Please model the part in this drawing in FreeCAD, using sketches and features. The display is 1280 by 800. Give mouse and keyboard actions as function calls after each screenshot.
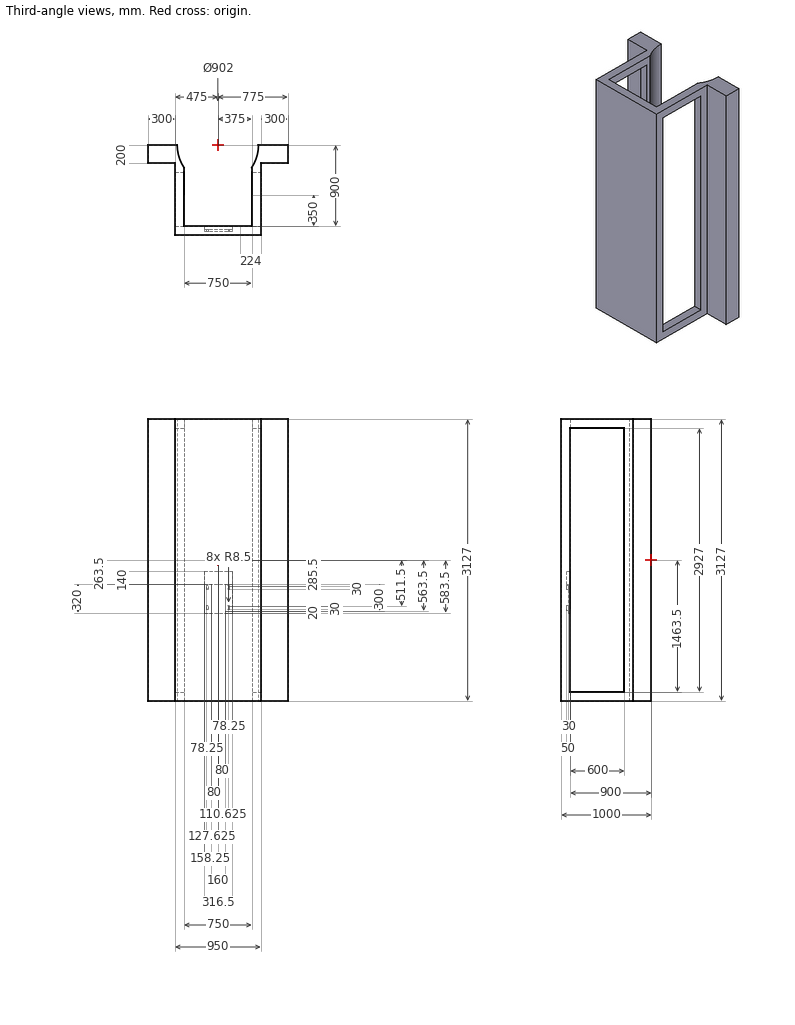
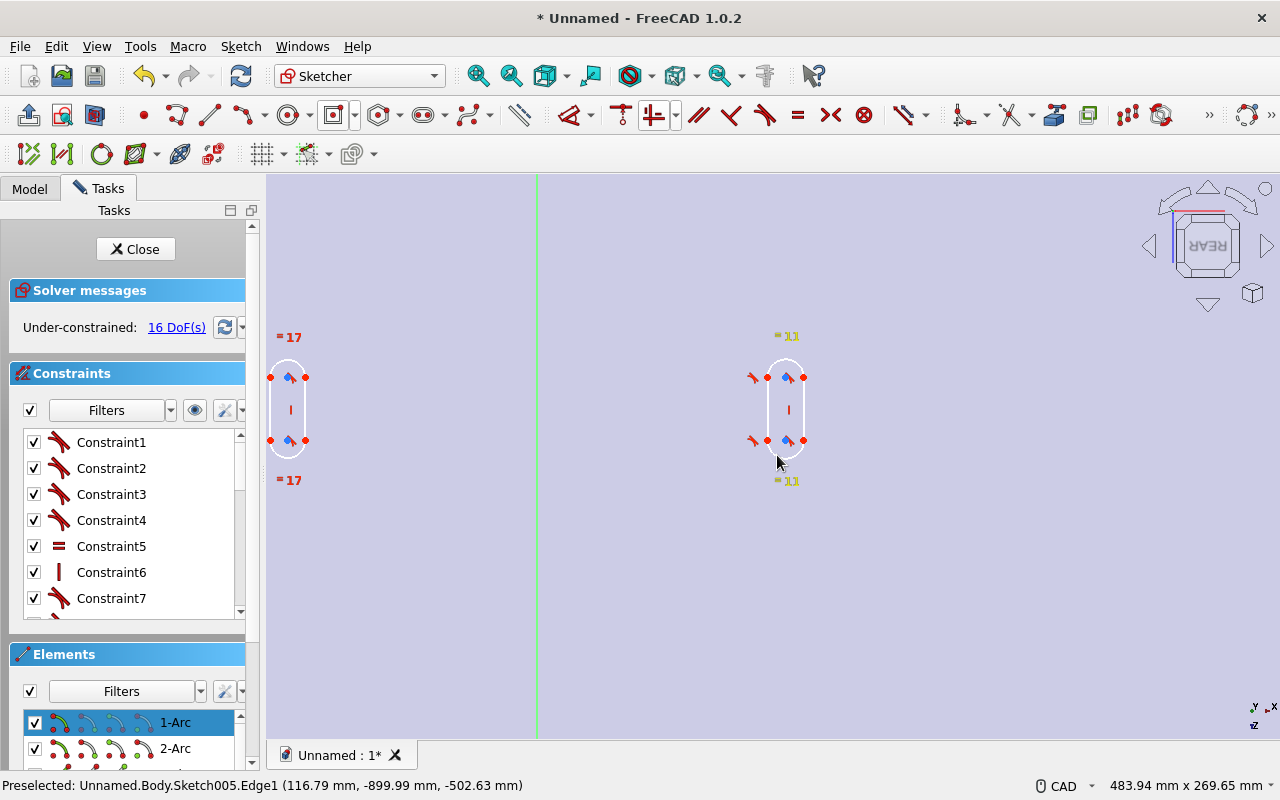
click(775, 455)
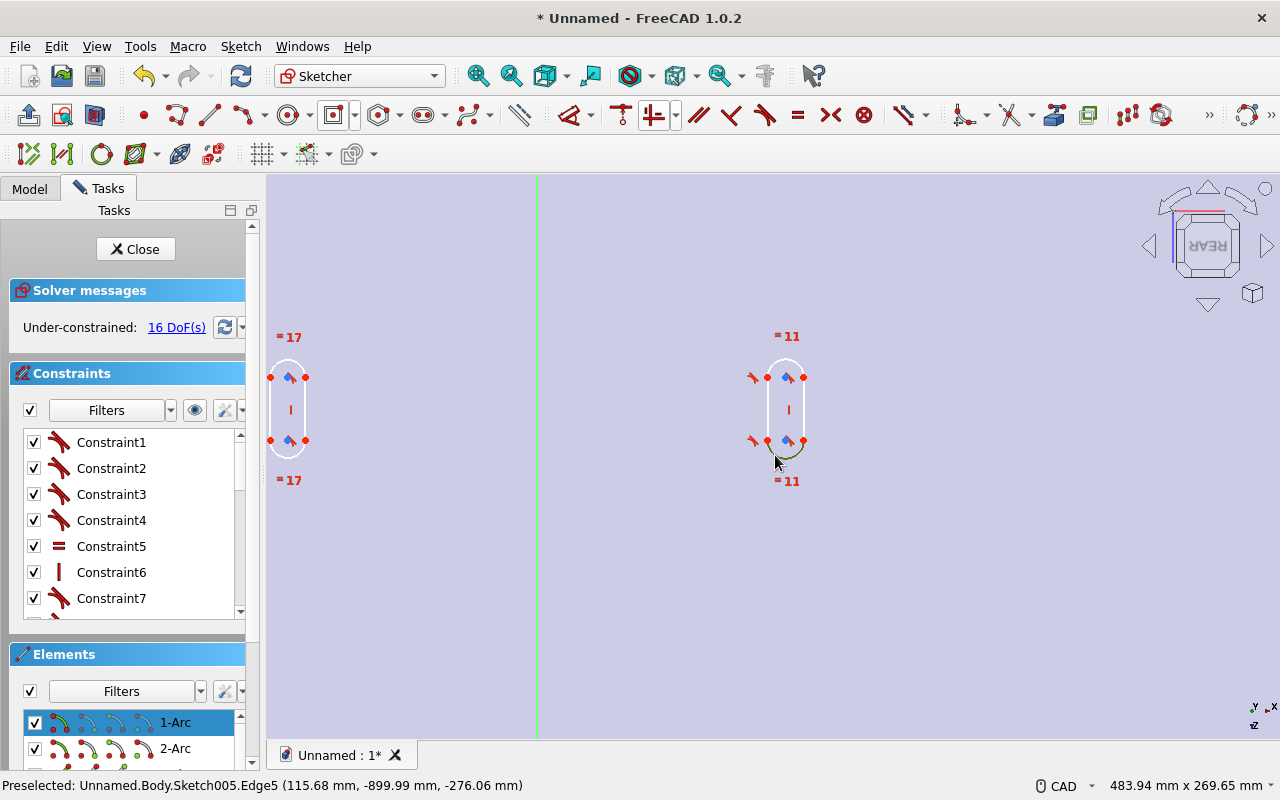
click(298, 455)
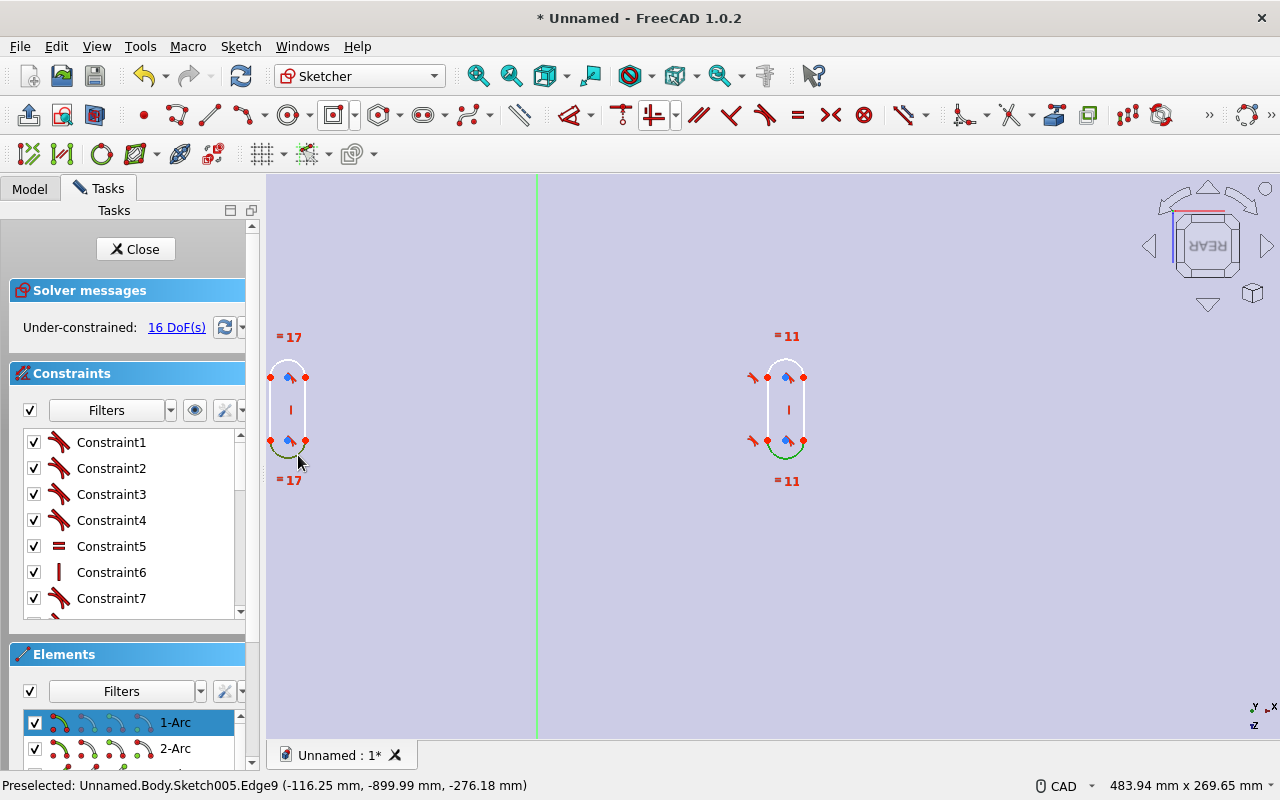
scroll(777, 455, down, 6)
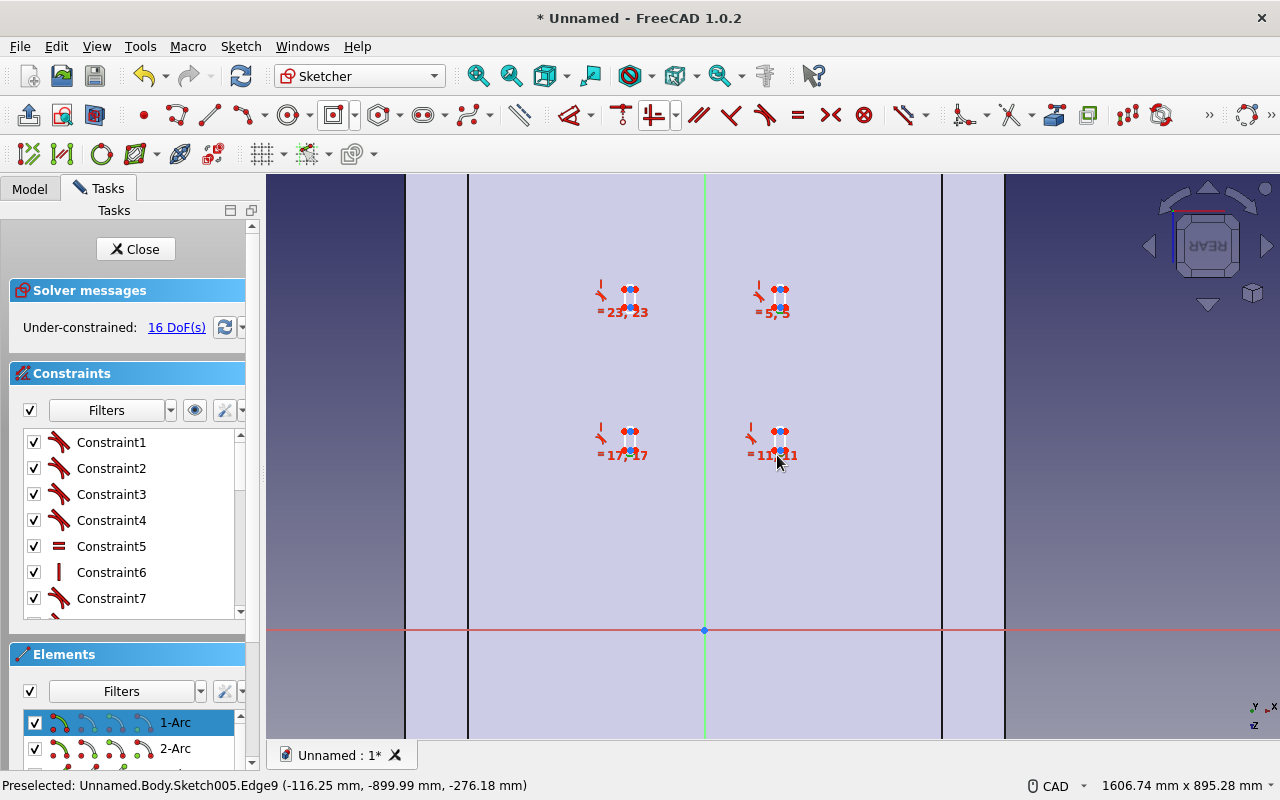
scroll(627, 312, up, 6)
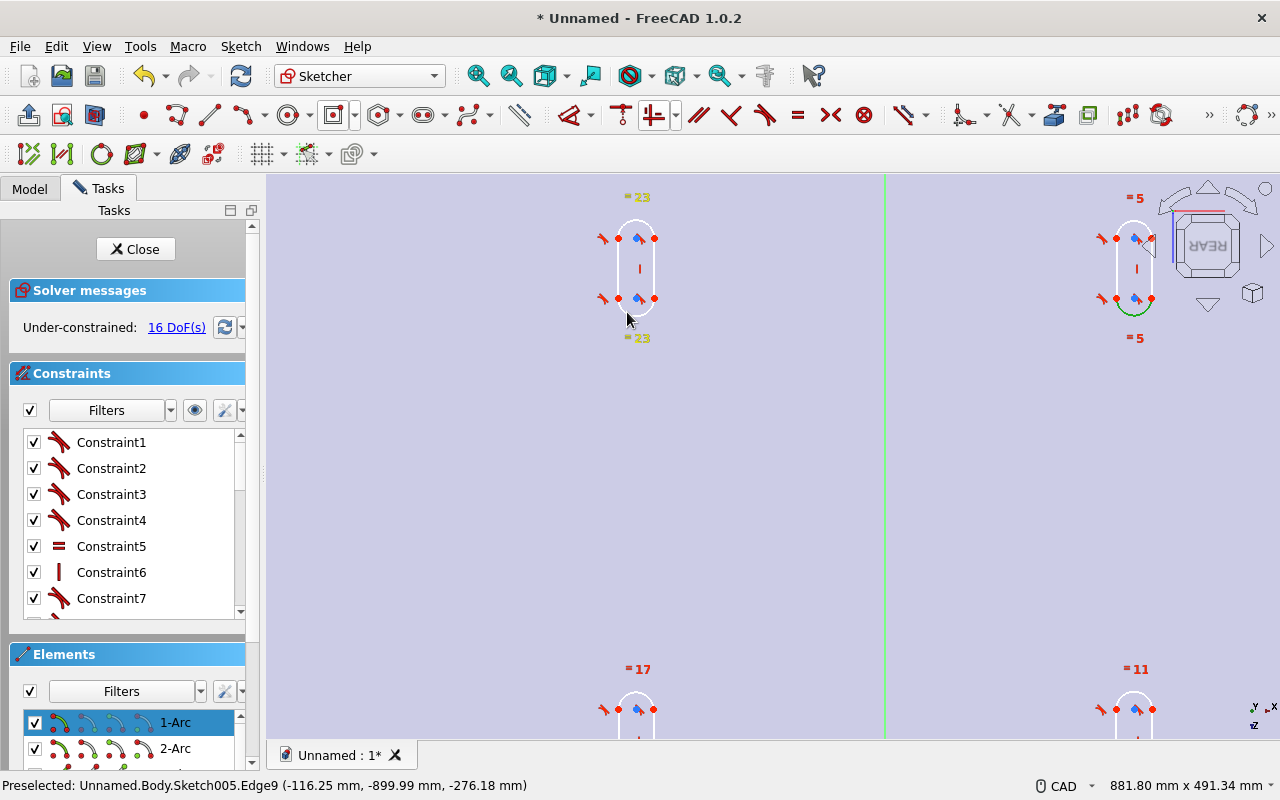
click(625, 313)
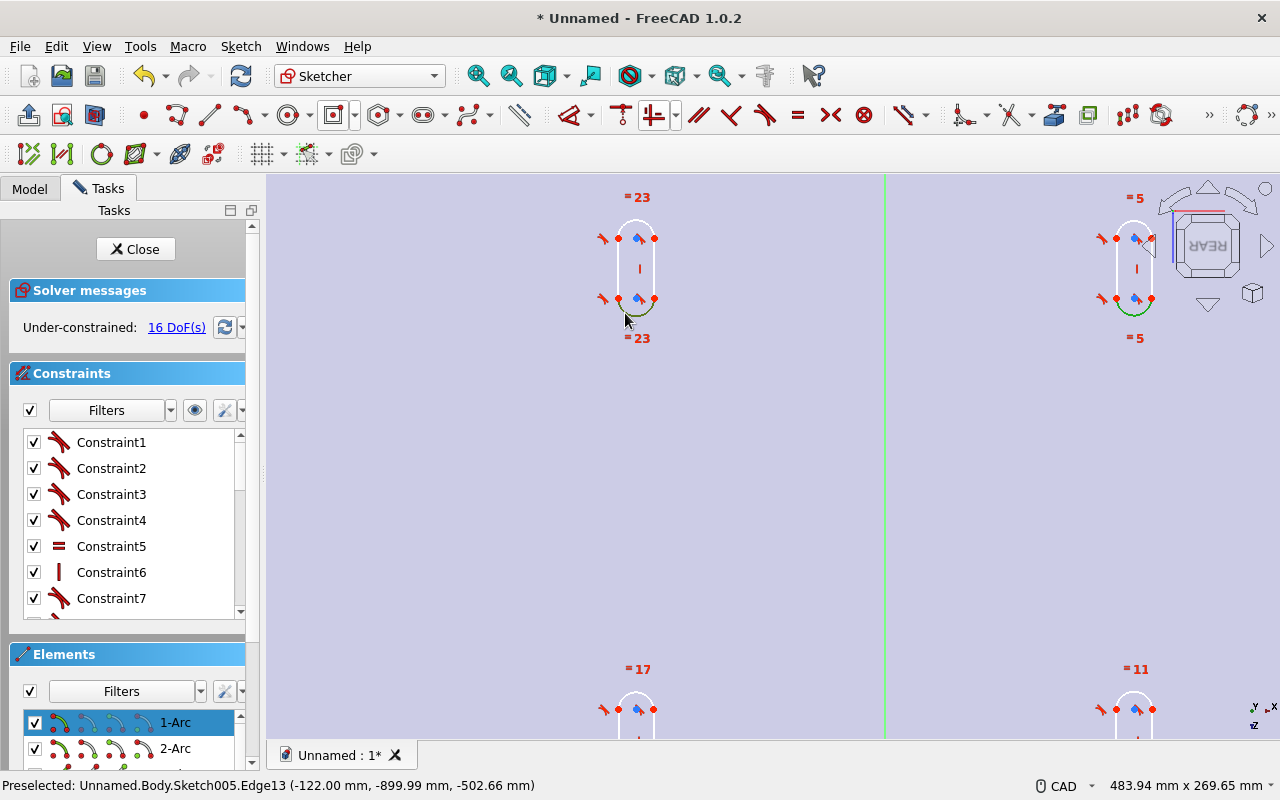
click(798, 116)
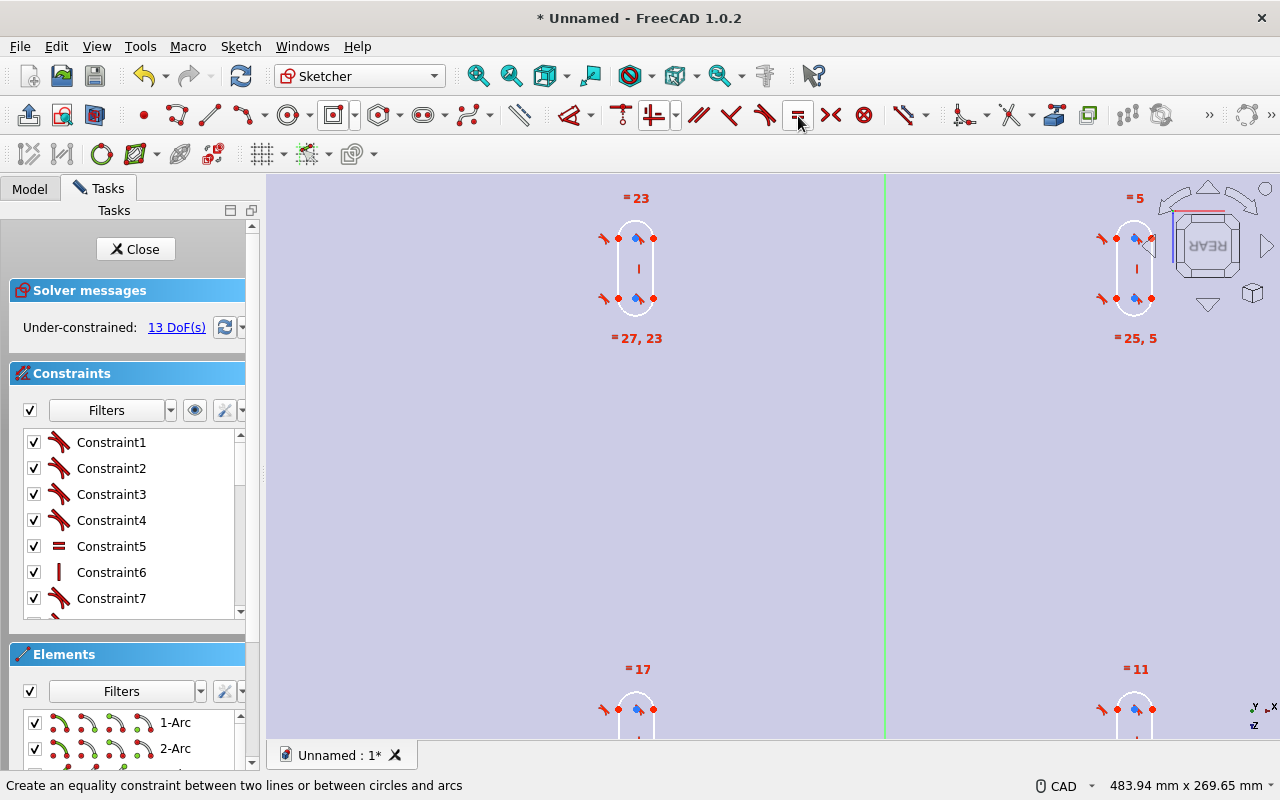
click(568, 116)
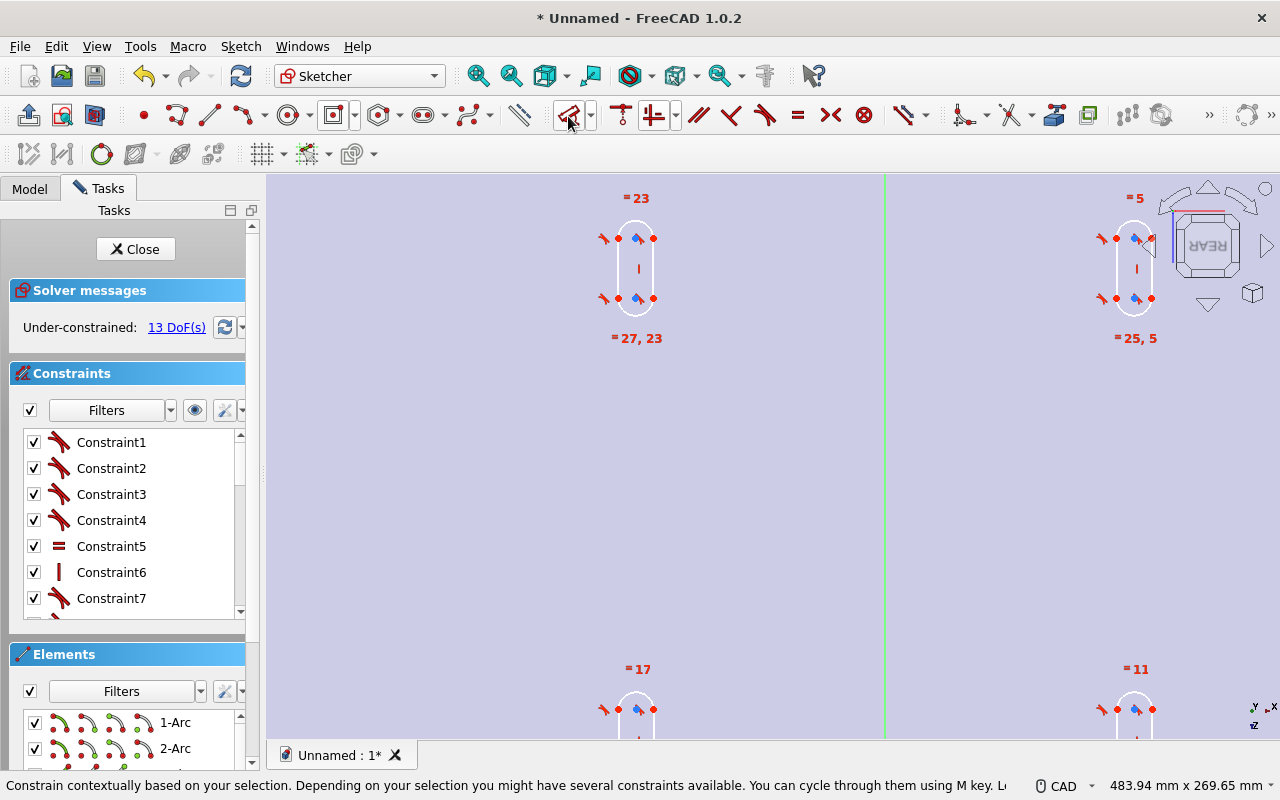
scroll(627, 312, down, 6)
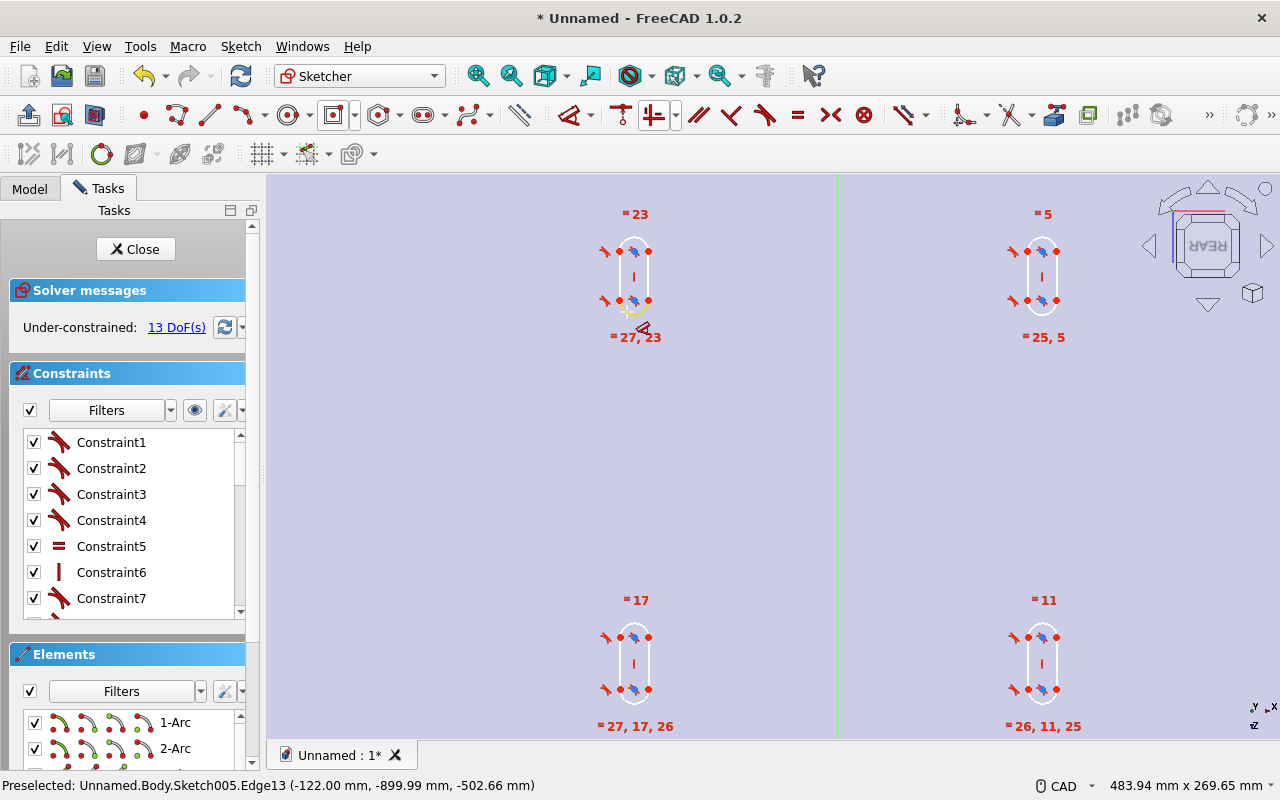
scroll(777, 312, up, 11)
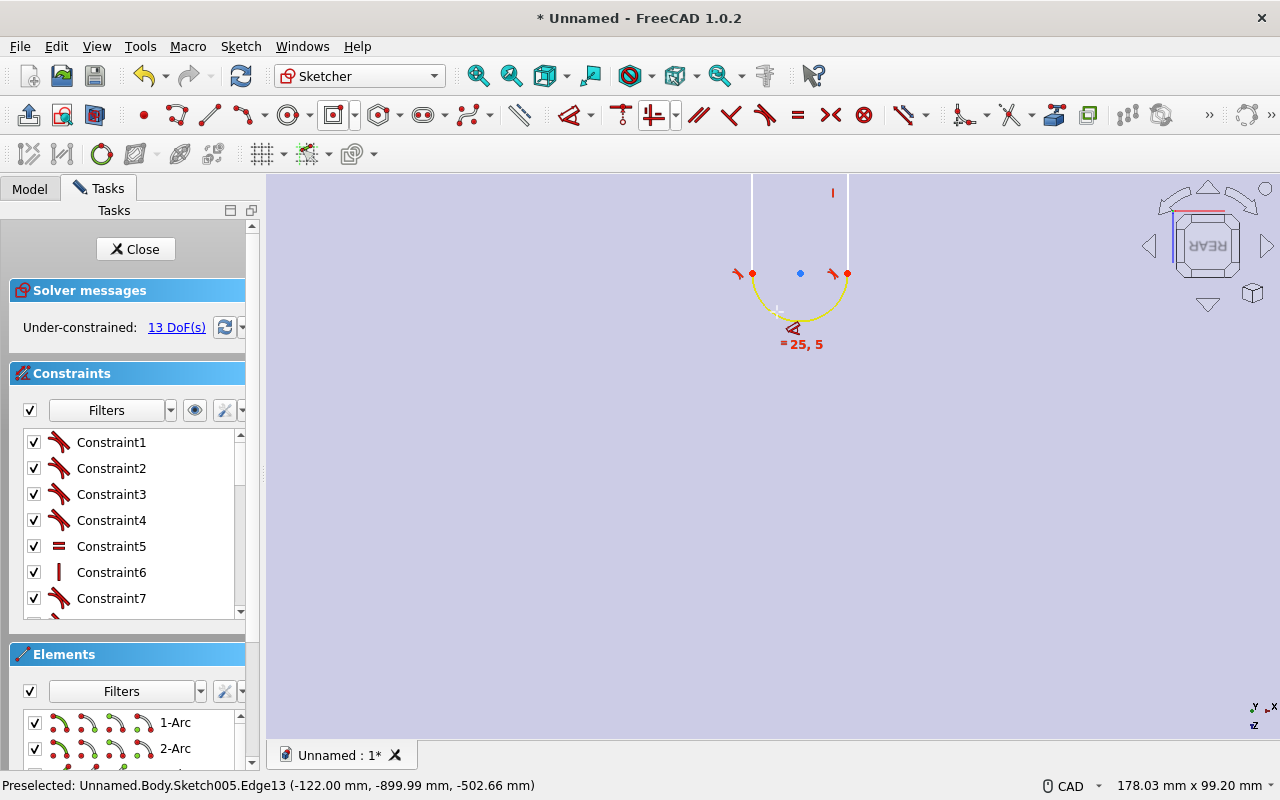
click(772, 312)
click(753, 338)